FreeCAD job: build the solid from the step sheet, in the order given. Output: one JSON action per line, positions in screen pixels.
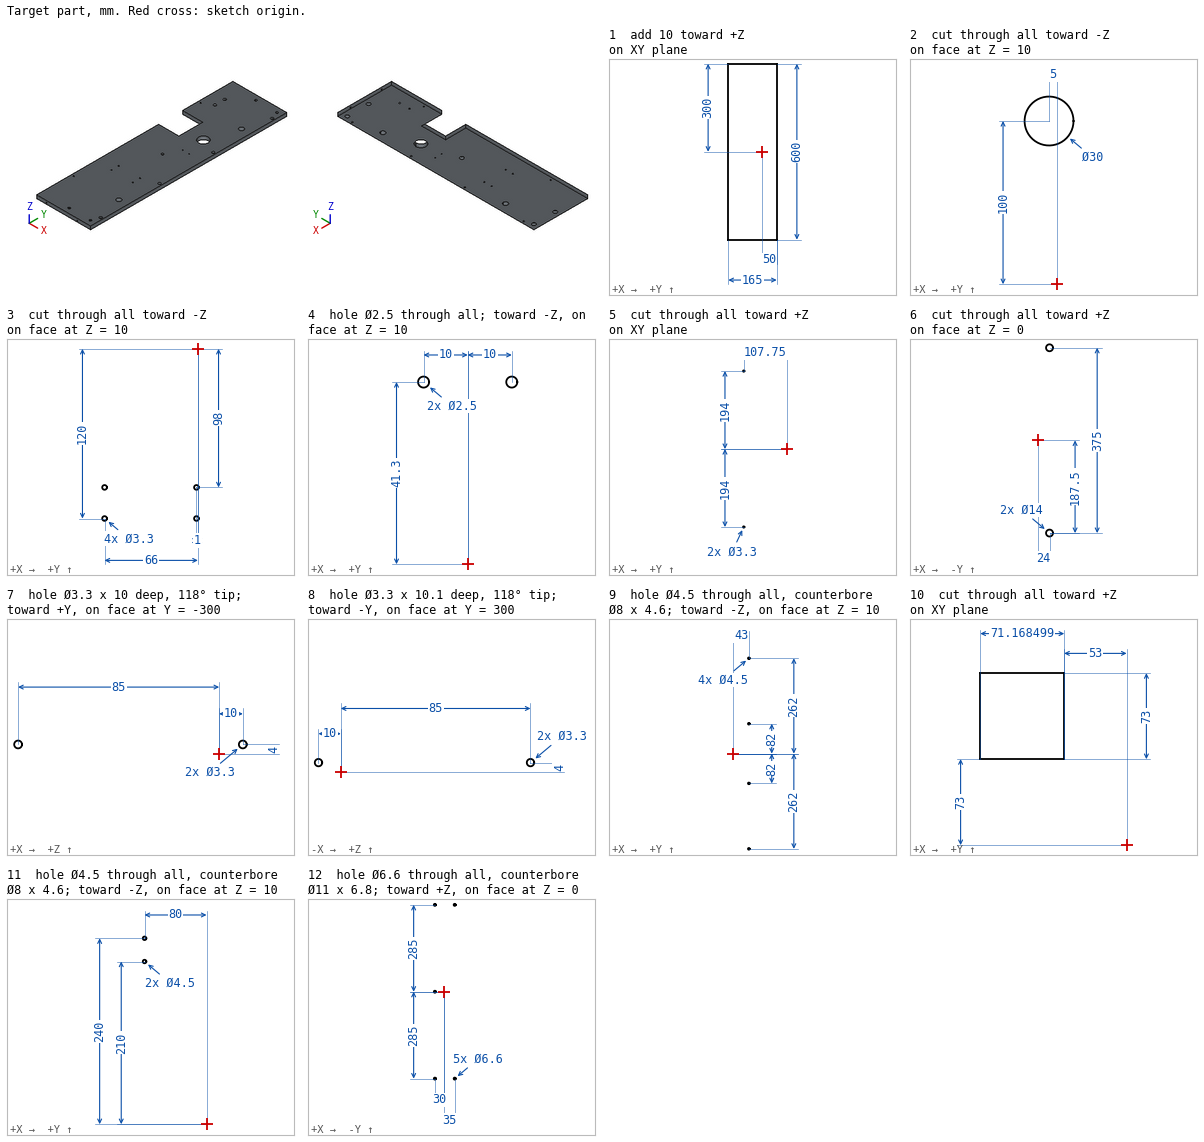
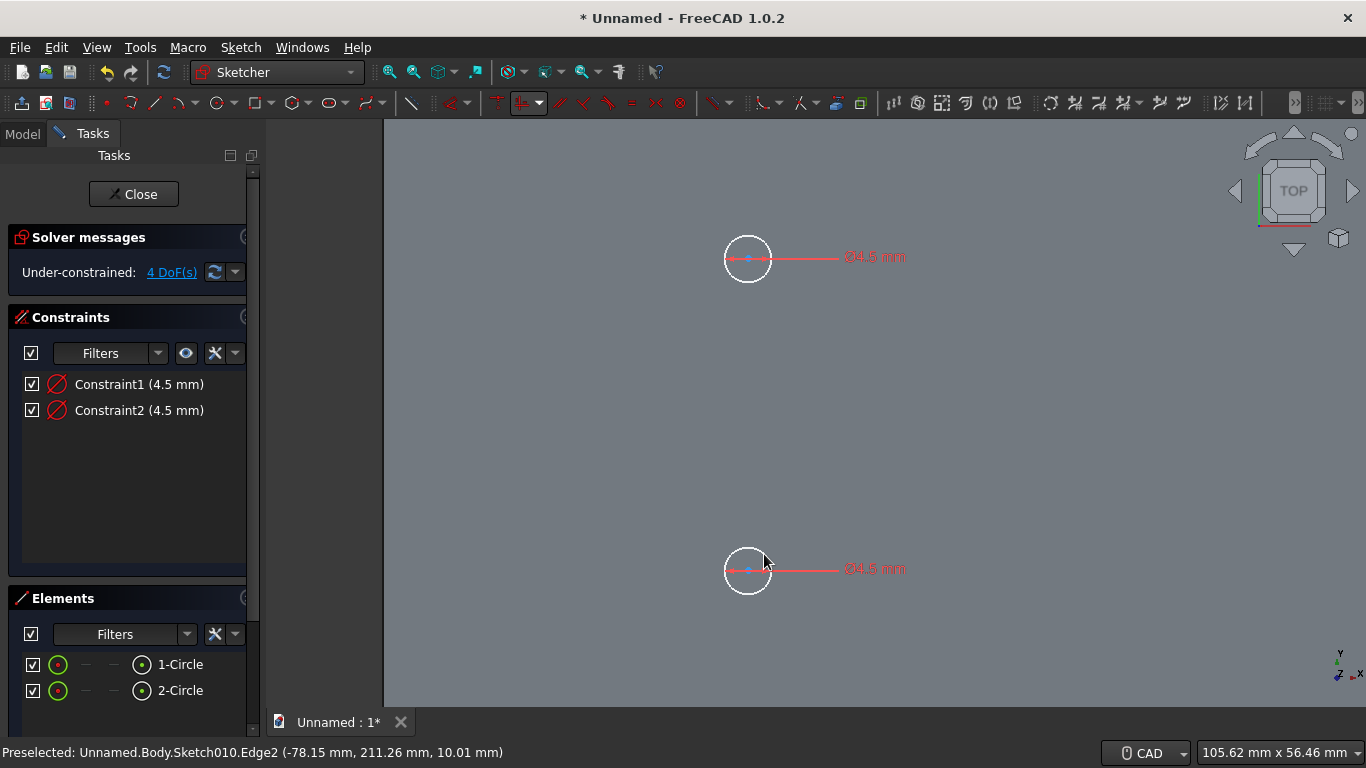
{"action": "left_click", "coordinate": [748, 259]}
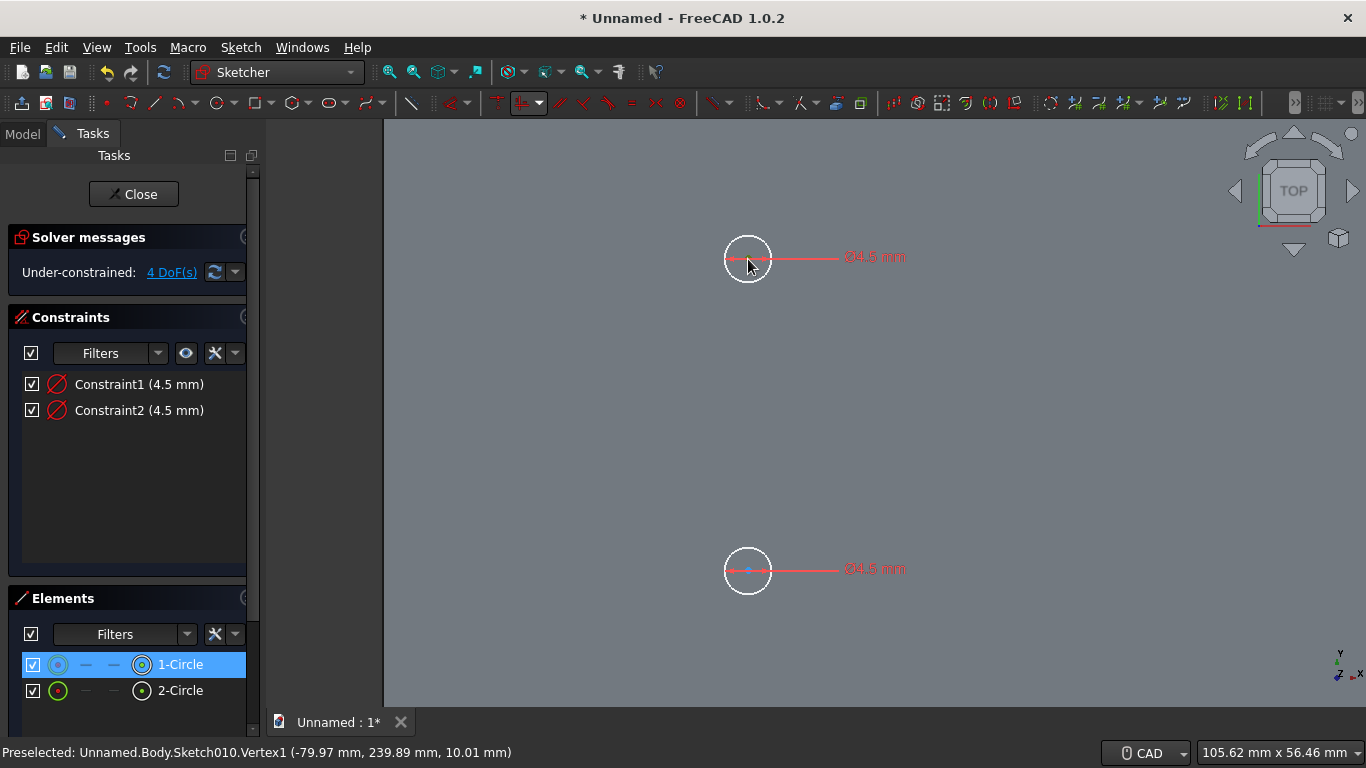
{"action": "left_click", "coordinate": [748, 571]}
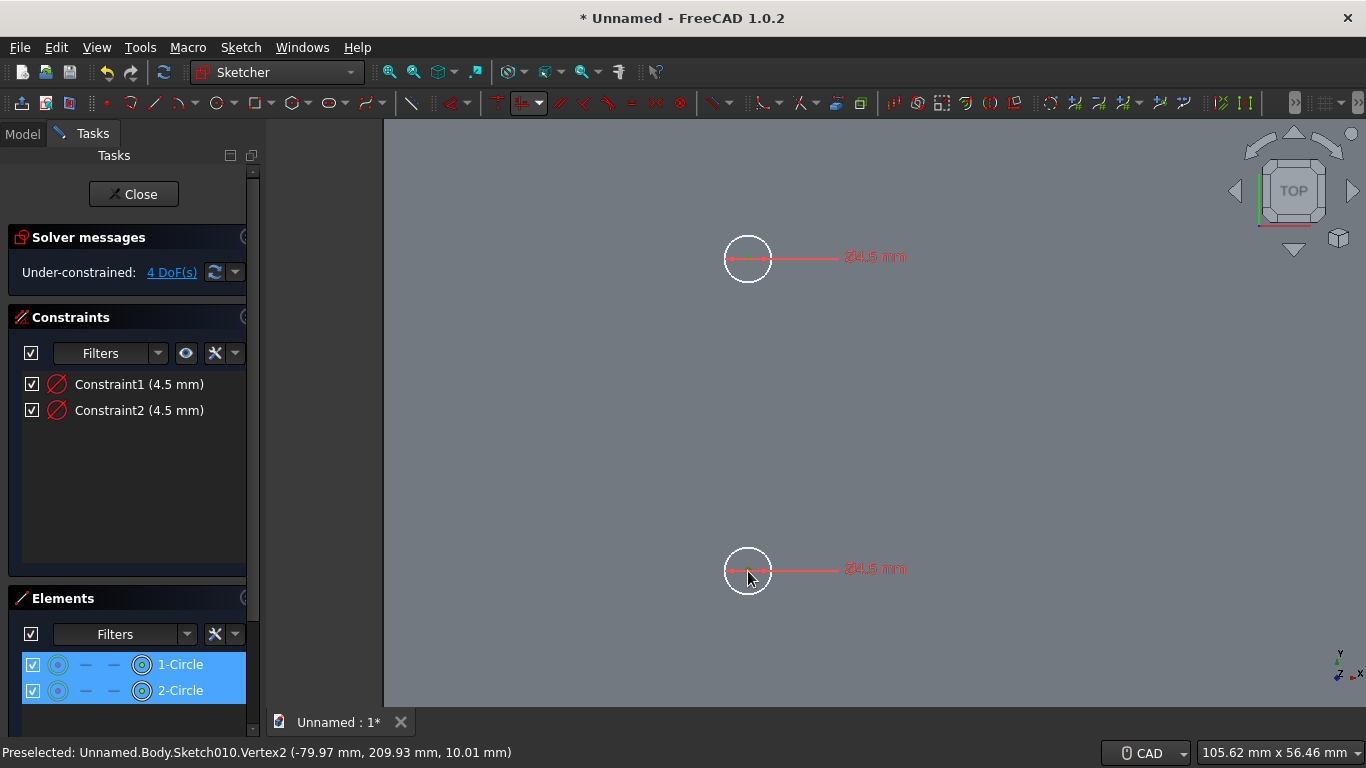
{"action": "left_click", "coordinate": [542, 104]}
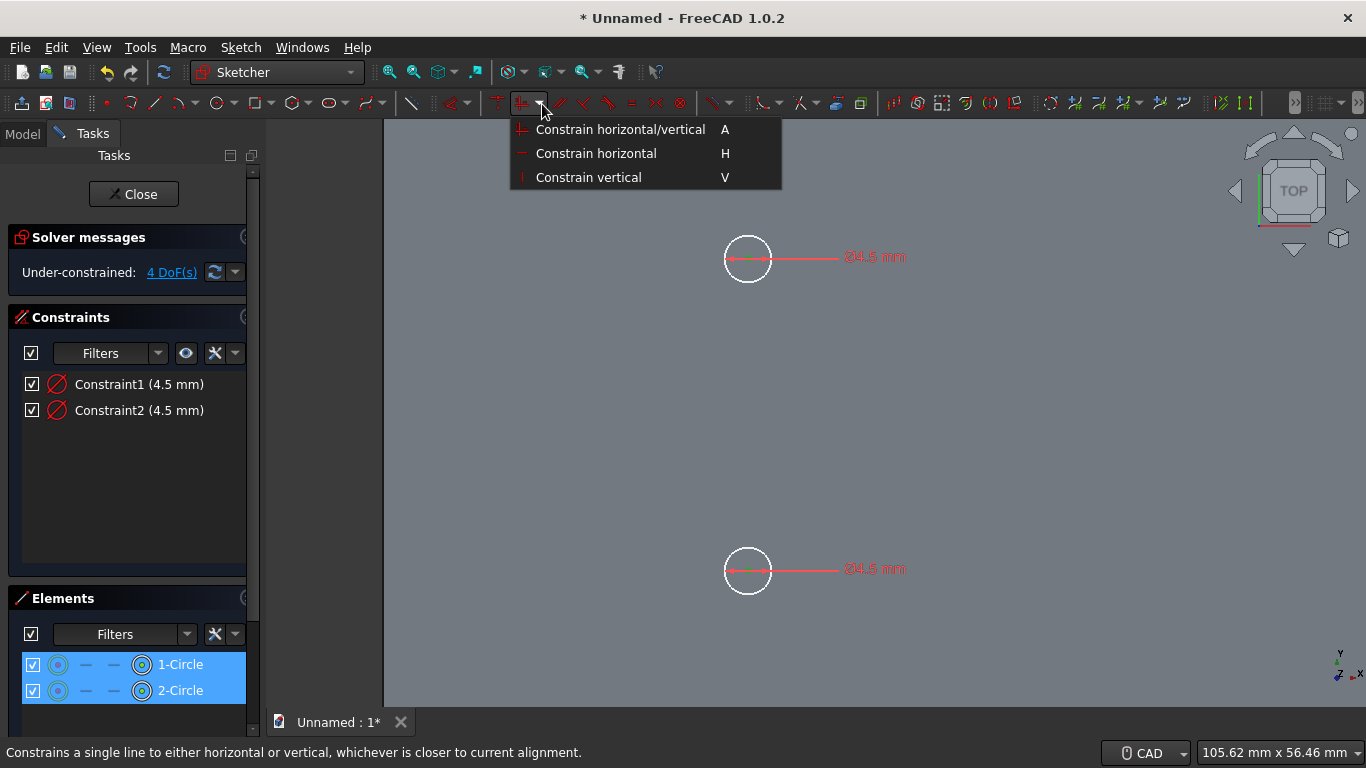
{"action": "left_click", "coordinate": [646, 177]}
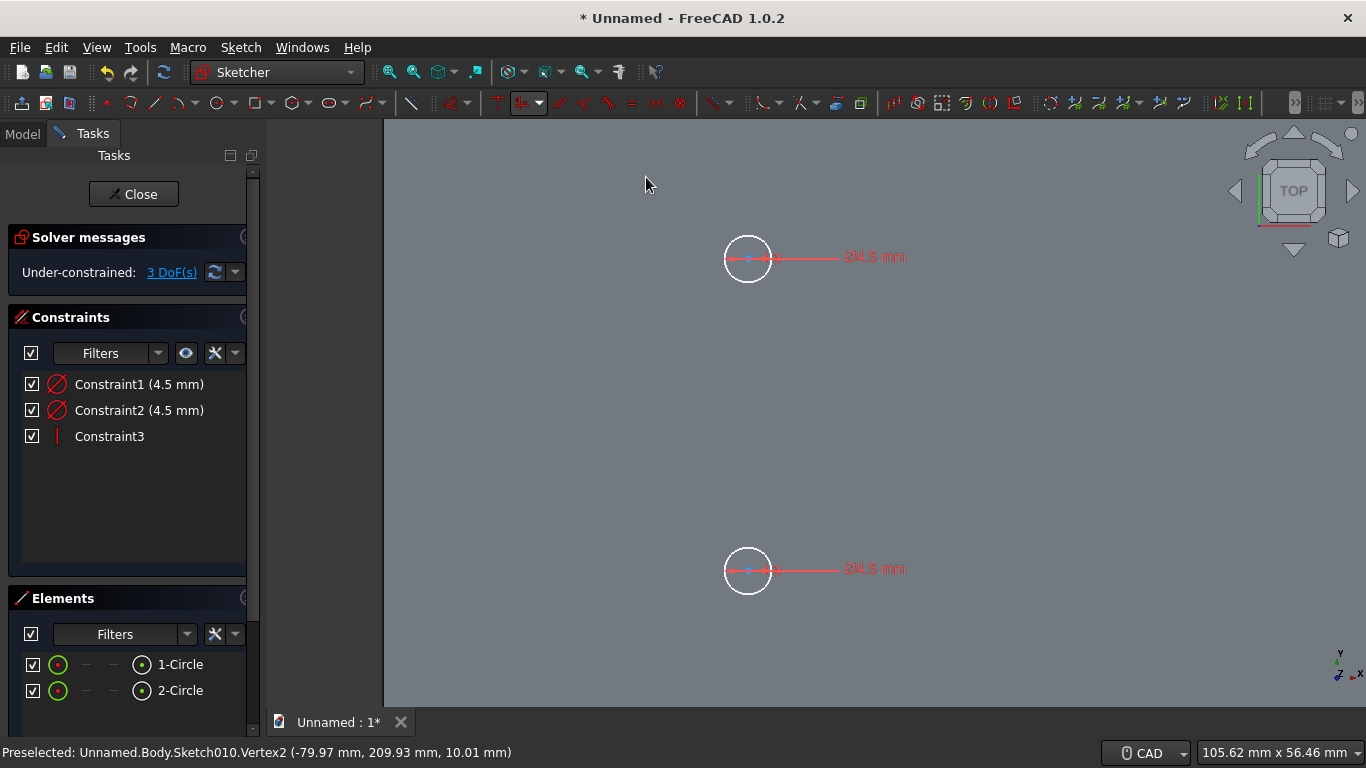
{"action": "left_click", "coordinate": [450, 104]}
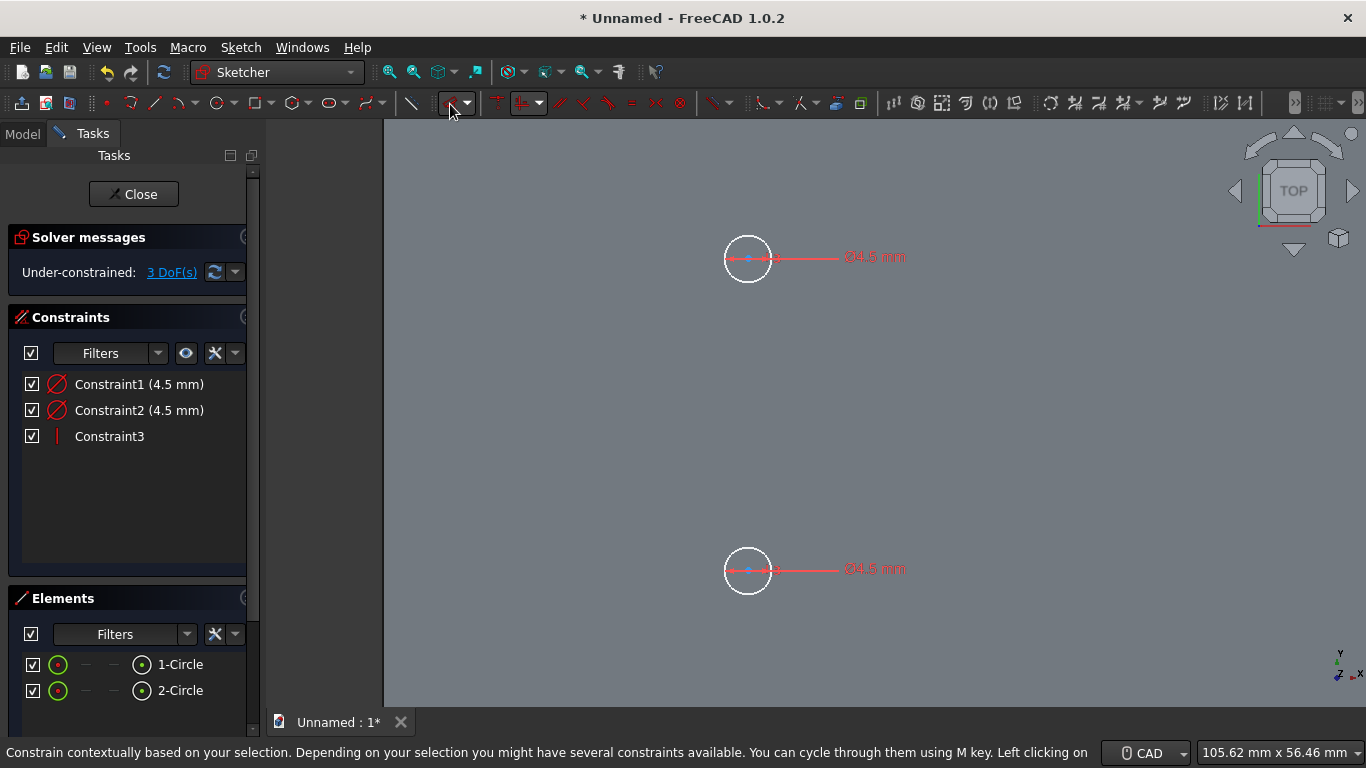
{"action": "left_click", "coordinate": [748, 259]}
{"action": "left_click", "coordinate": [974, 225]}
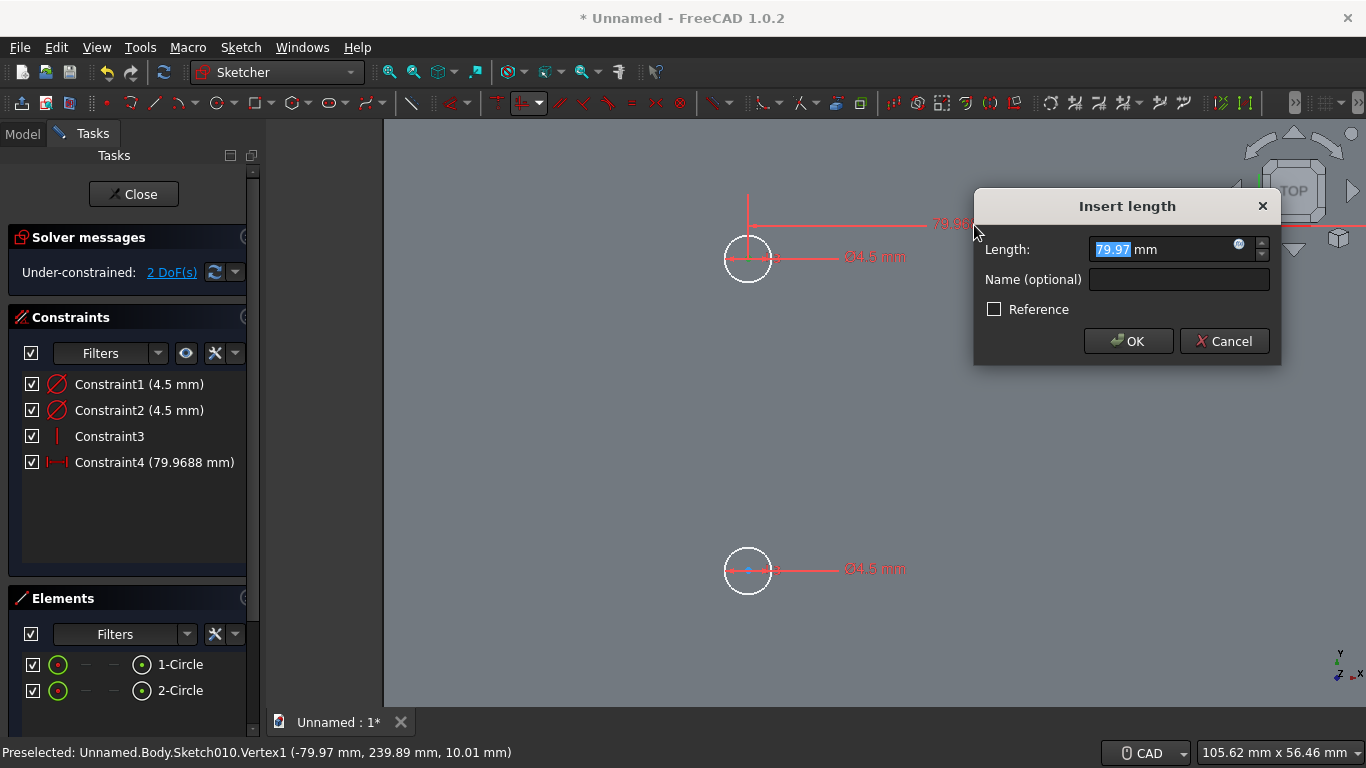
{"action": "type", "text": "80"}
{"action": "key", "text": "Return"}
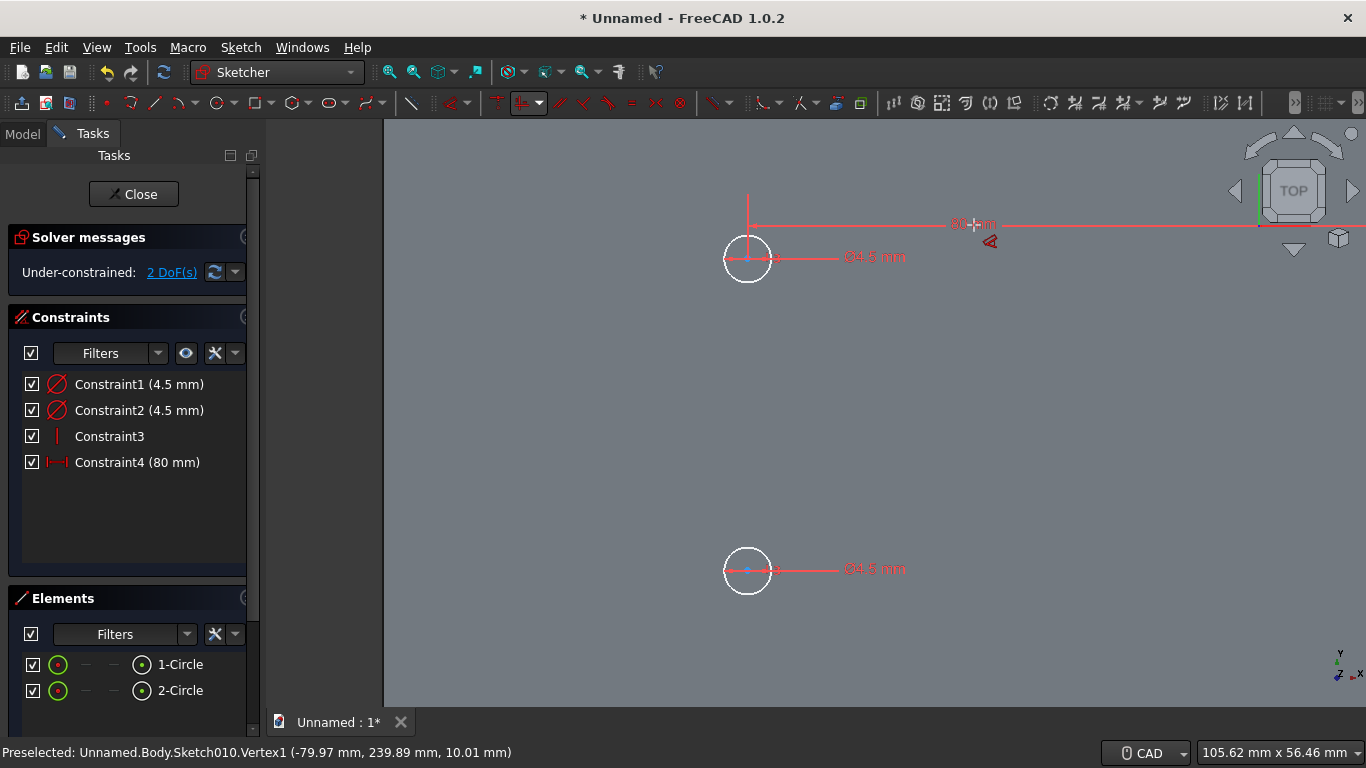
{"action": "left_click", "coordinate": [748, 259]}
{"action": "left_click", "coordinate": [714, 469]}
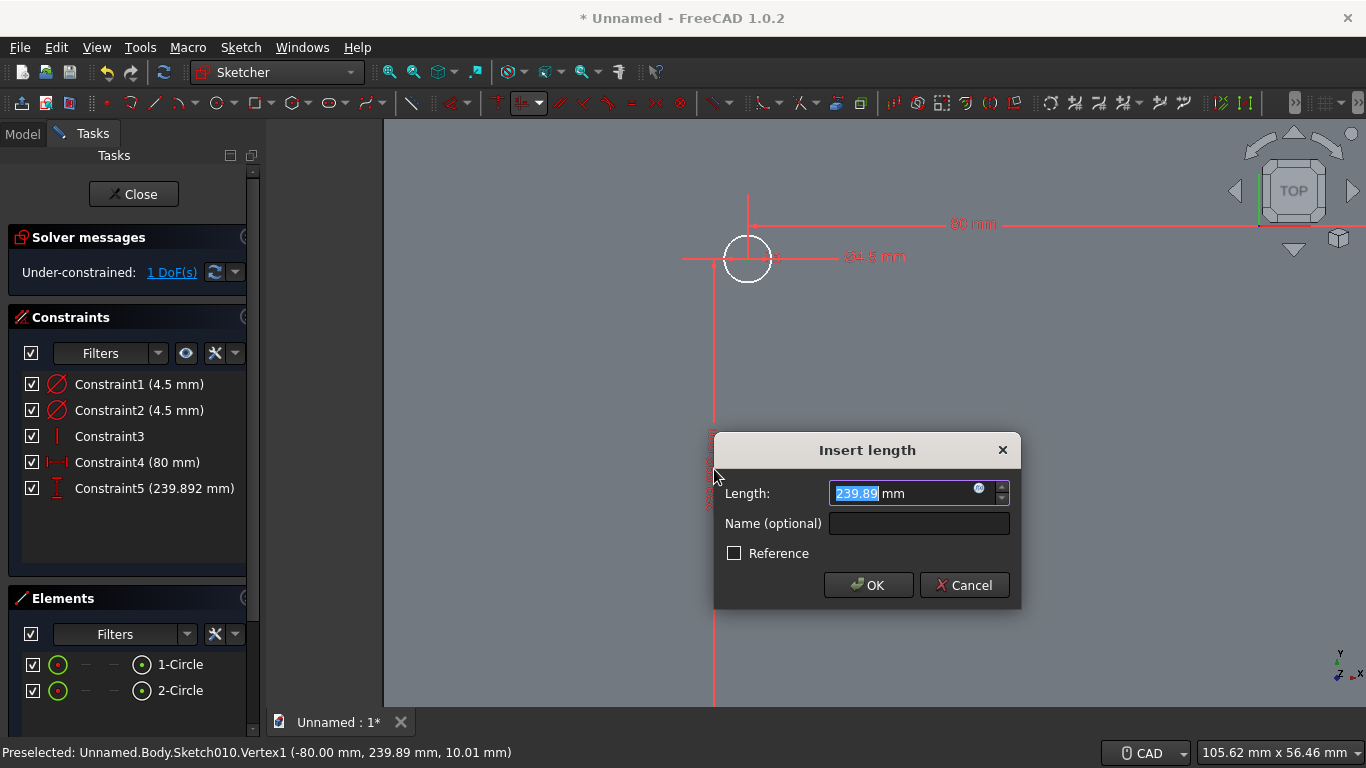
{"action": "type", "text": "240"}
{"action": "key", "text": "Return"}